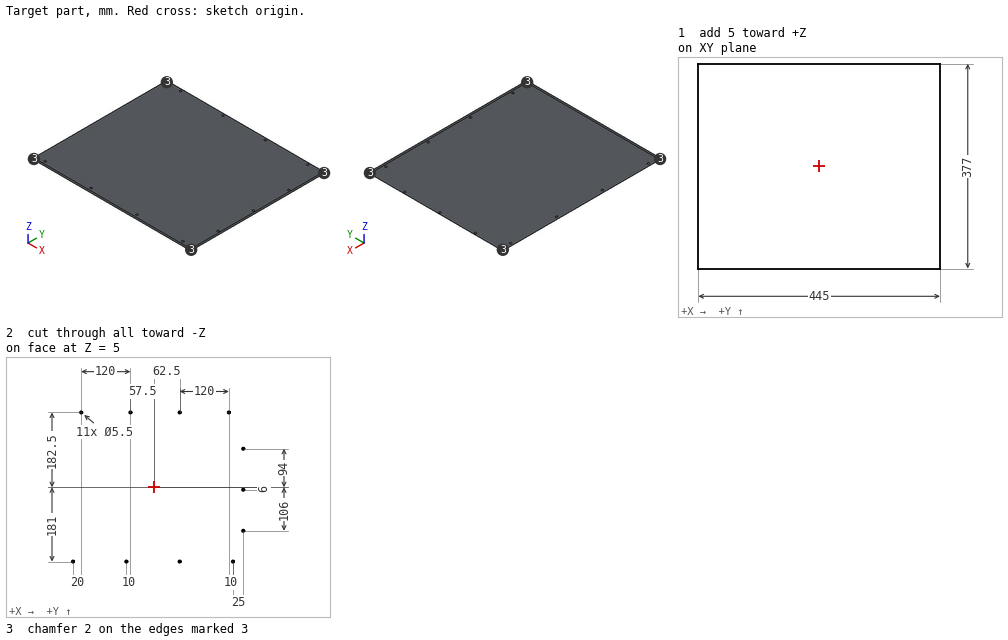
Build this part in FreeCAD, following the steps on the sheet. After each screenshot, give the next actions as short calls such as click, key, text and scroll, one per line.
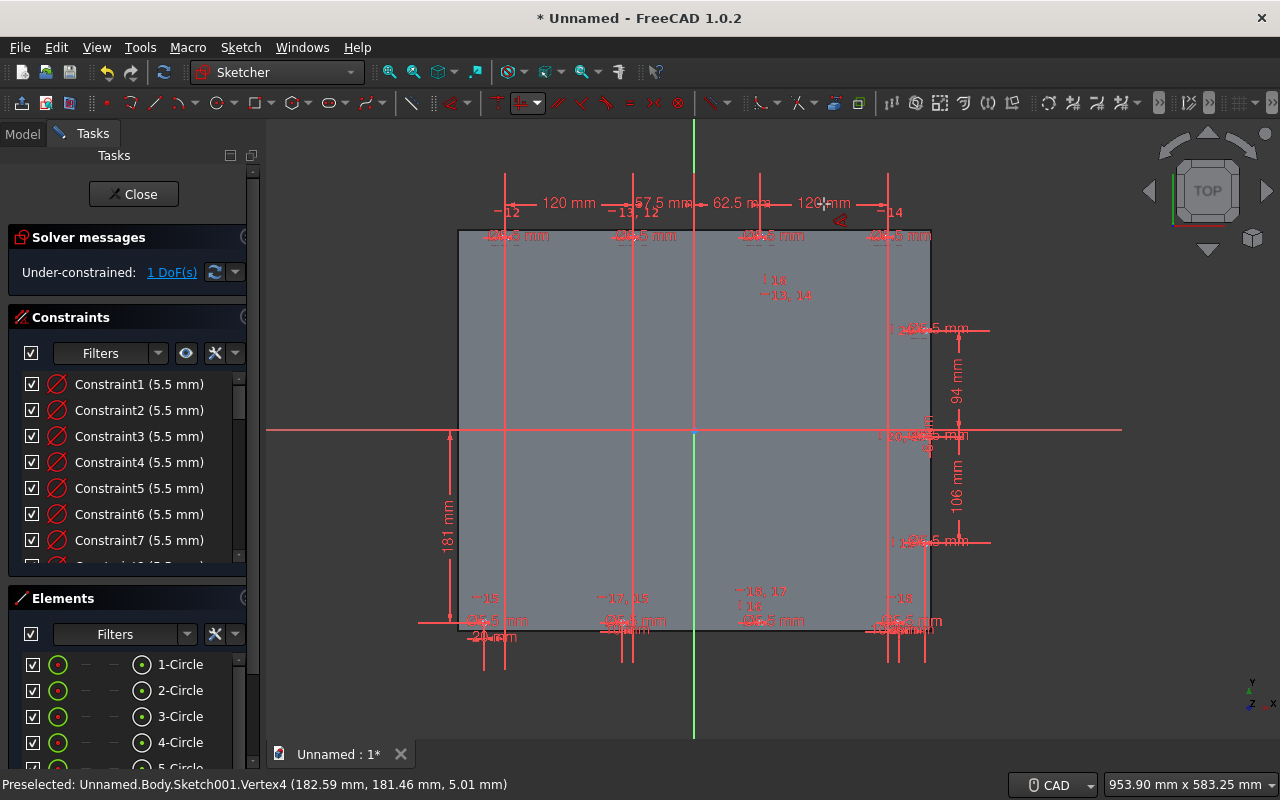
click(505, 238)
click(471, 334)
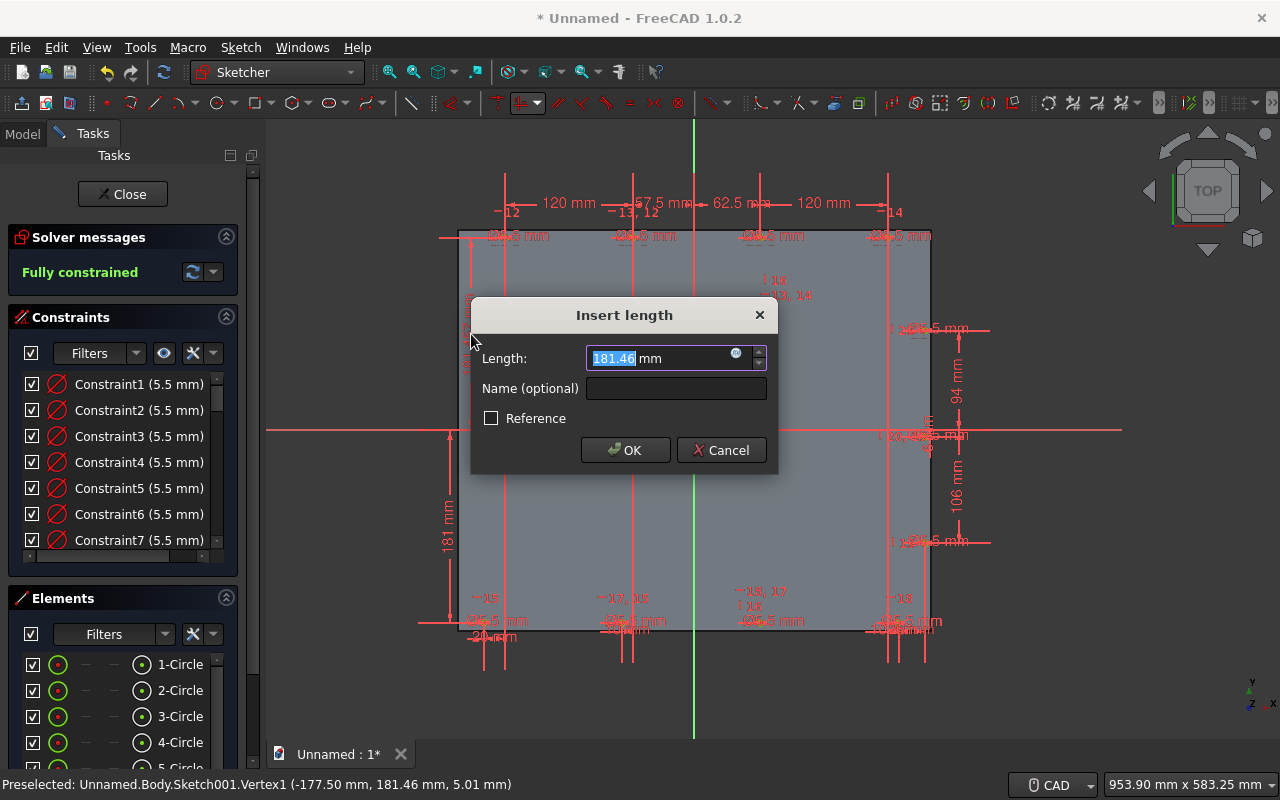
text(182.5)
key(Return)
key(Escape)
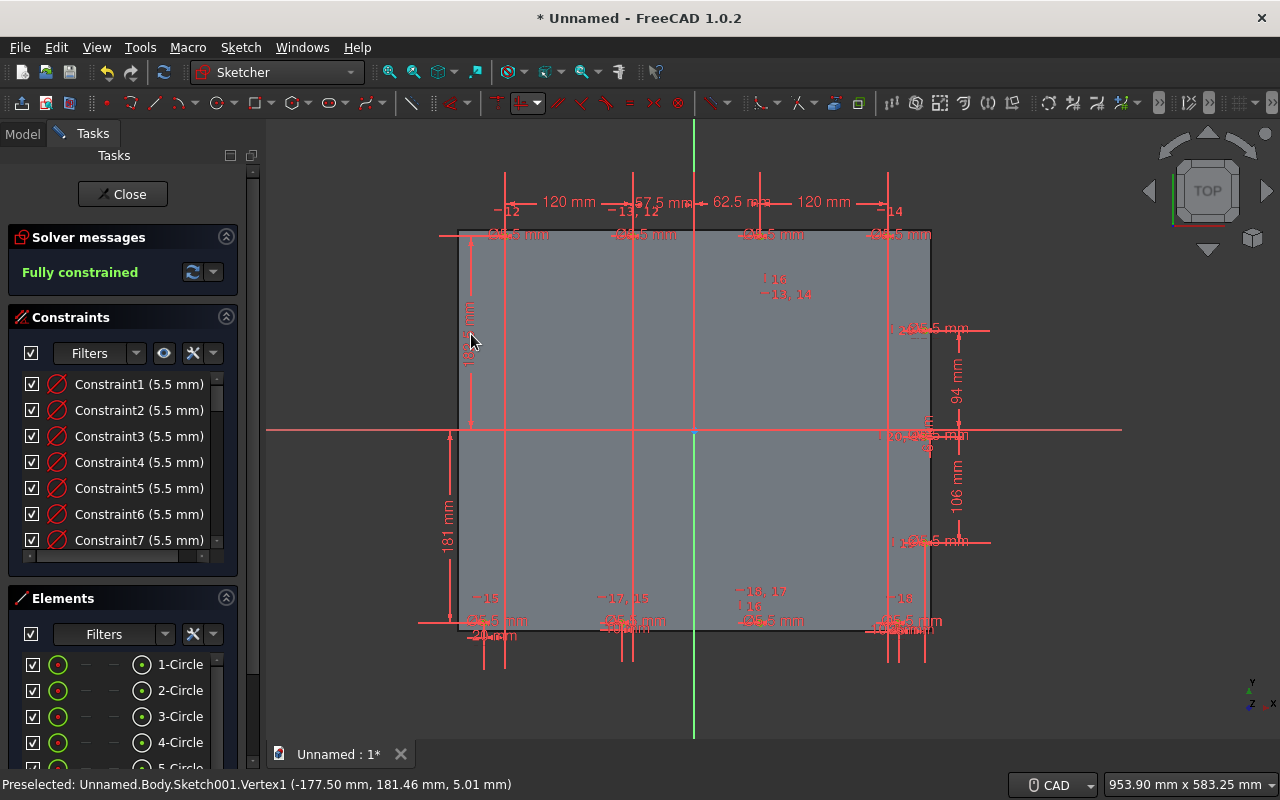
click(123, 194)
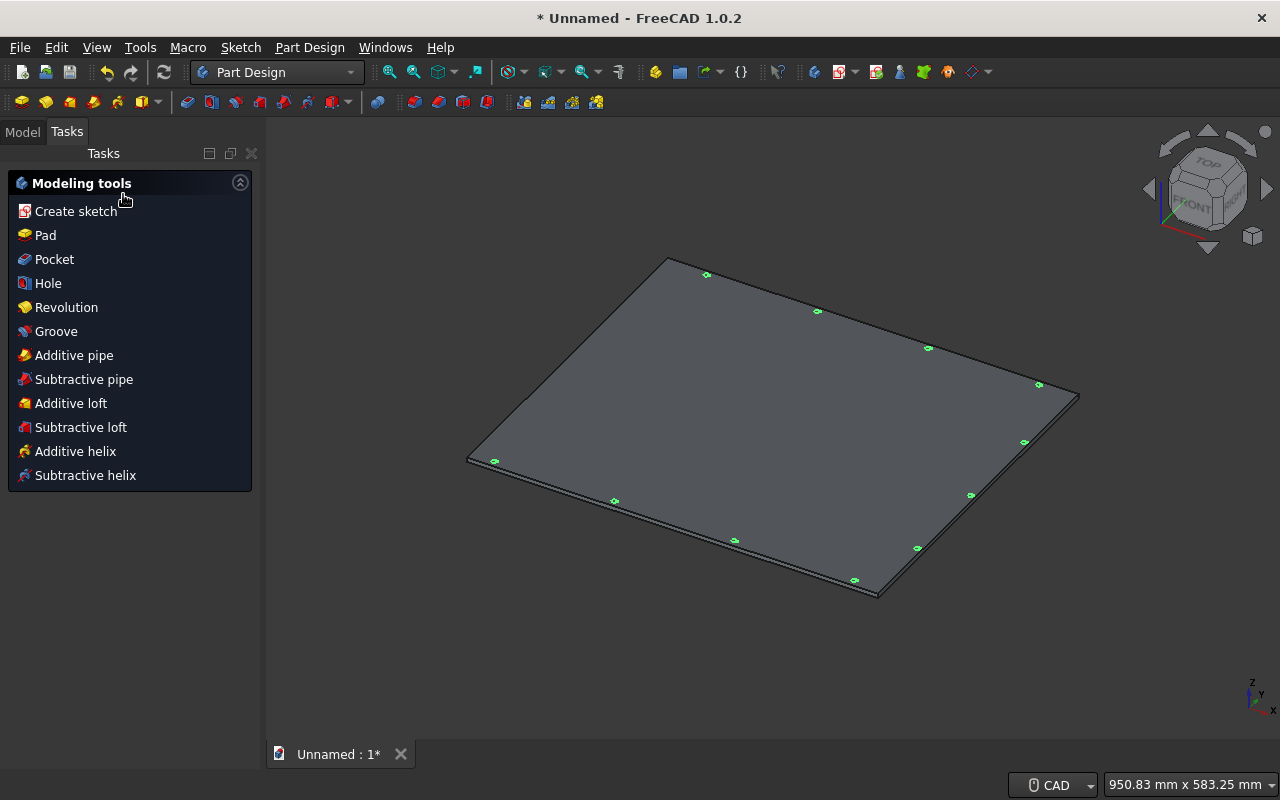
click(188, 102)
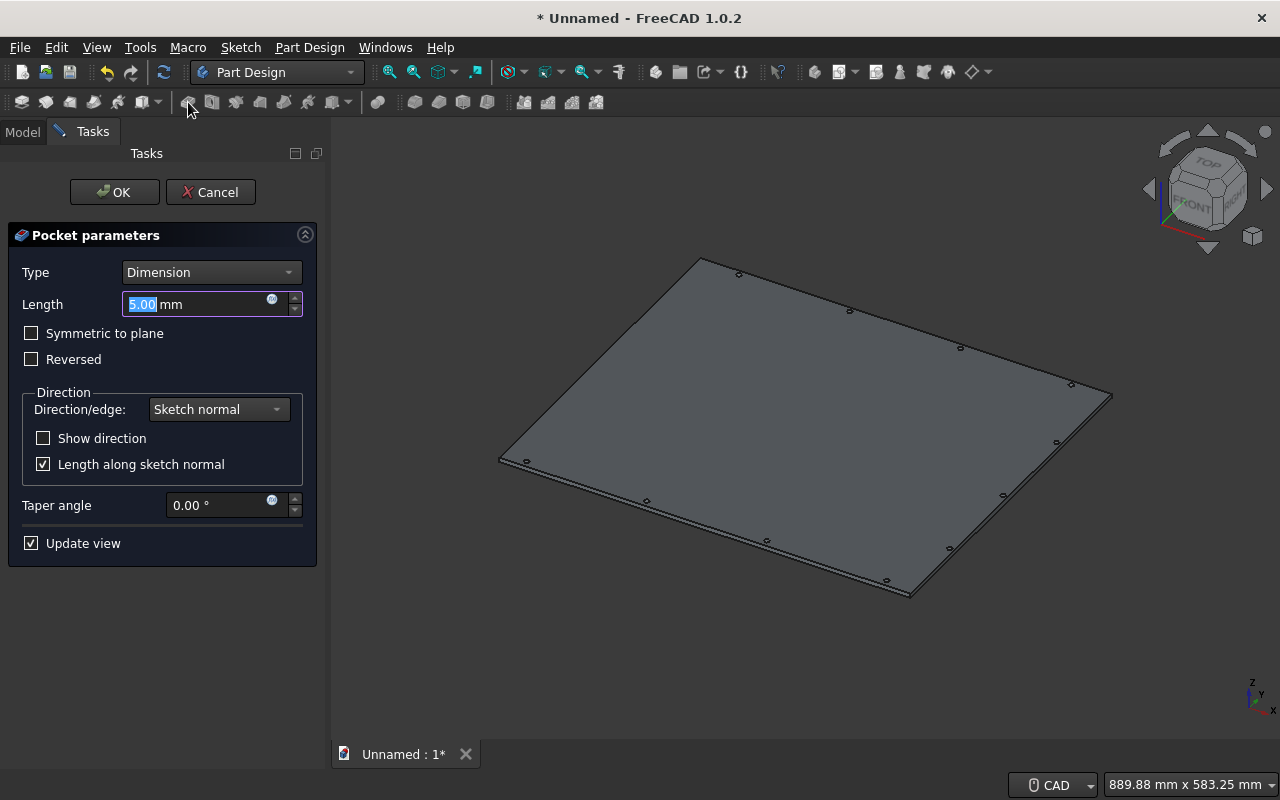
click(212, 272)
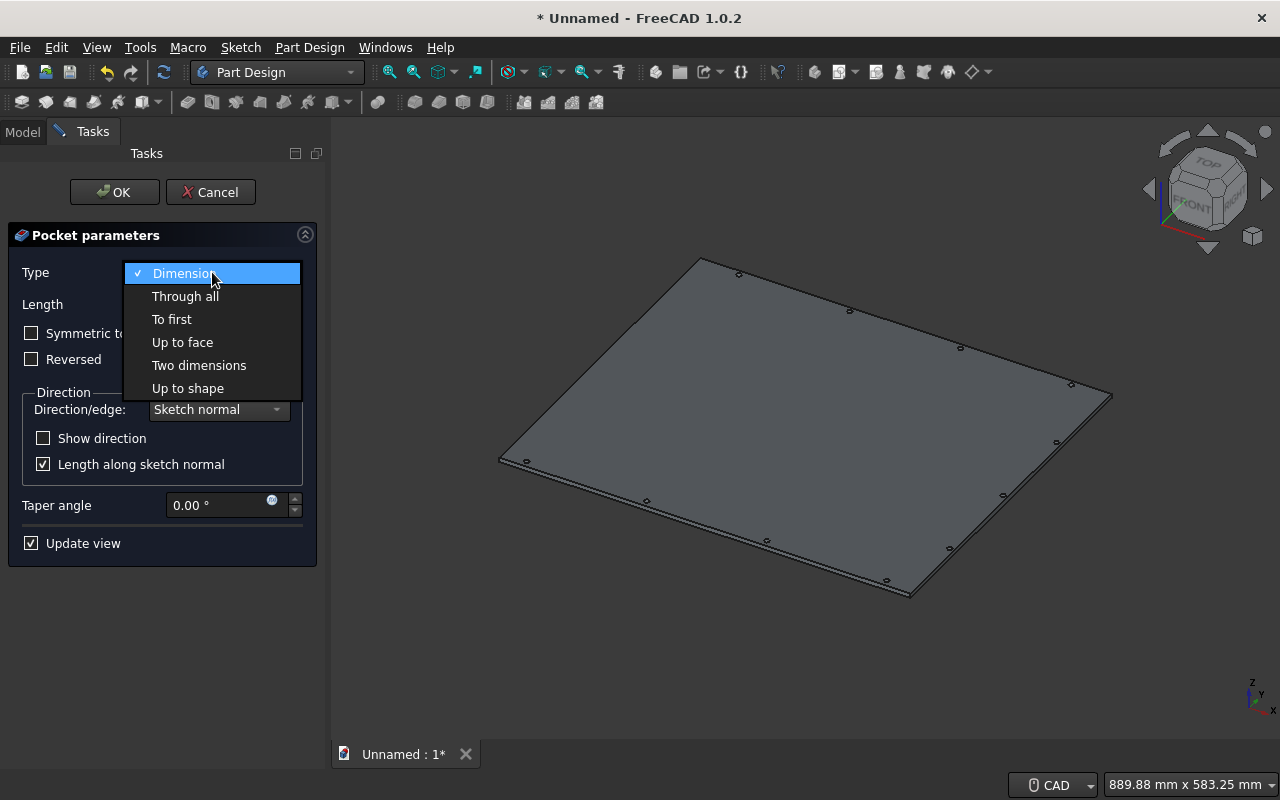
click(212, 296)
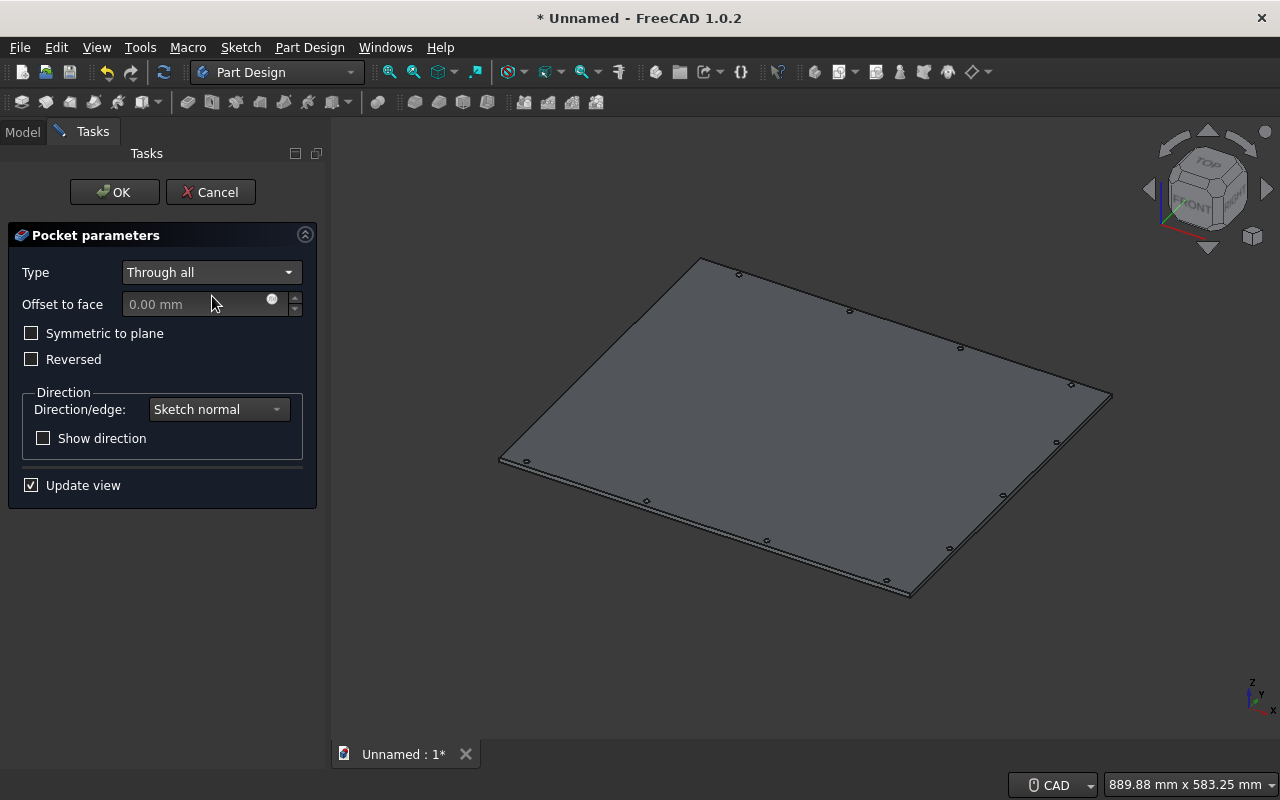
click(115, 192)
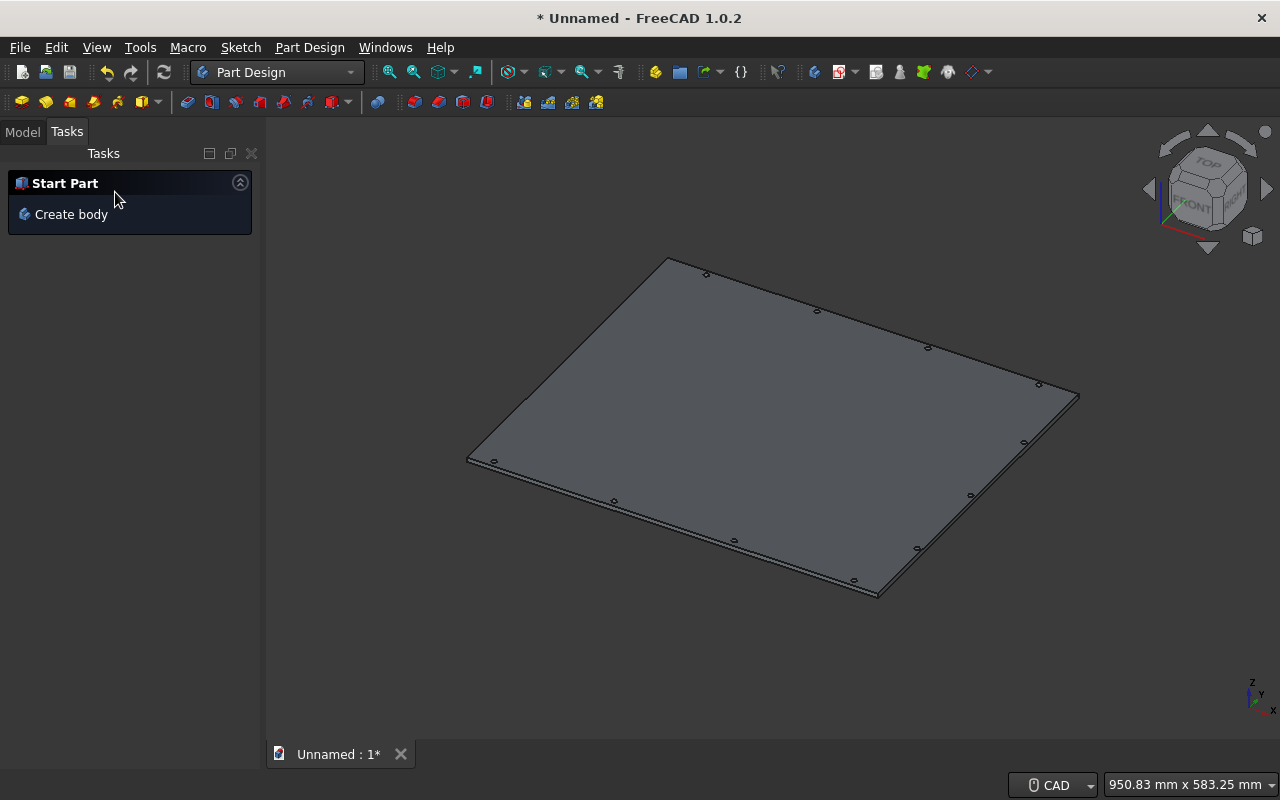
scroll(878, 595, up, 11)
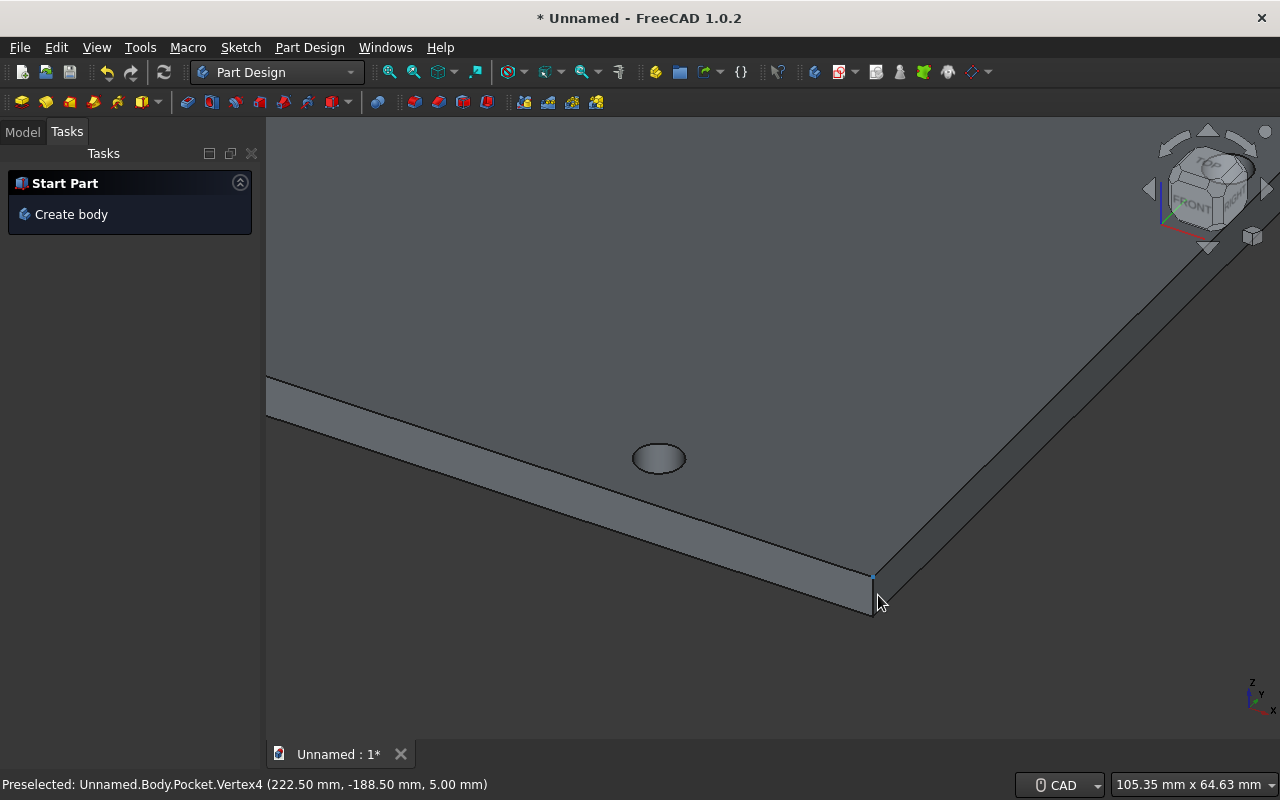
click(873, 596)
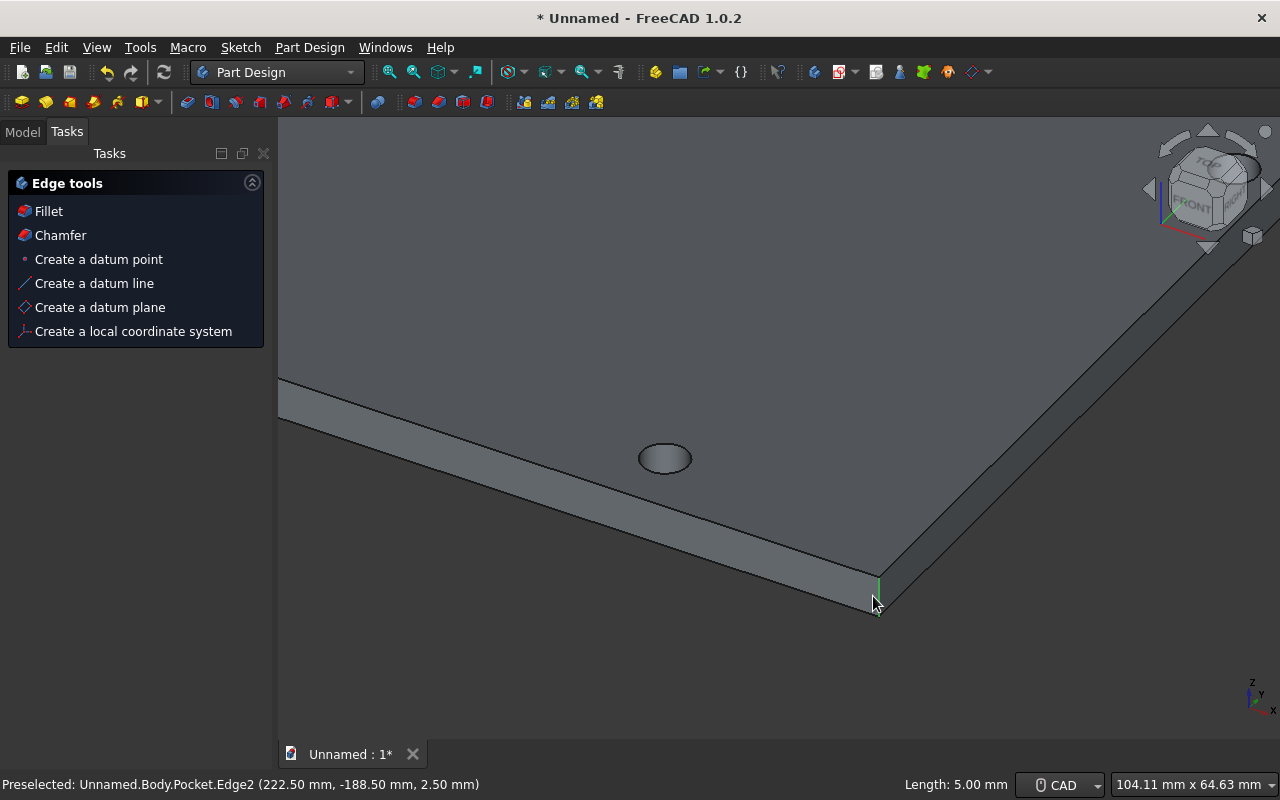
click(390, 72)